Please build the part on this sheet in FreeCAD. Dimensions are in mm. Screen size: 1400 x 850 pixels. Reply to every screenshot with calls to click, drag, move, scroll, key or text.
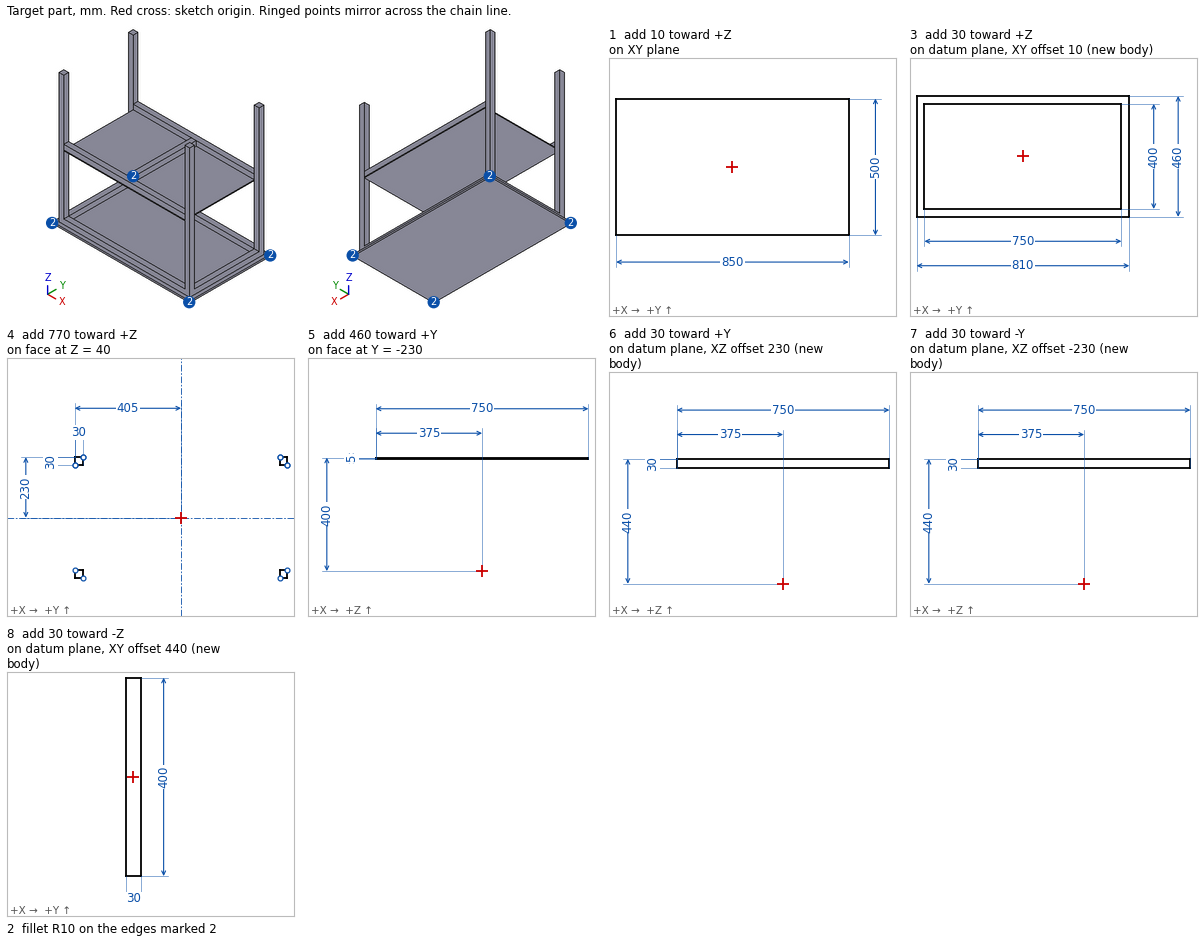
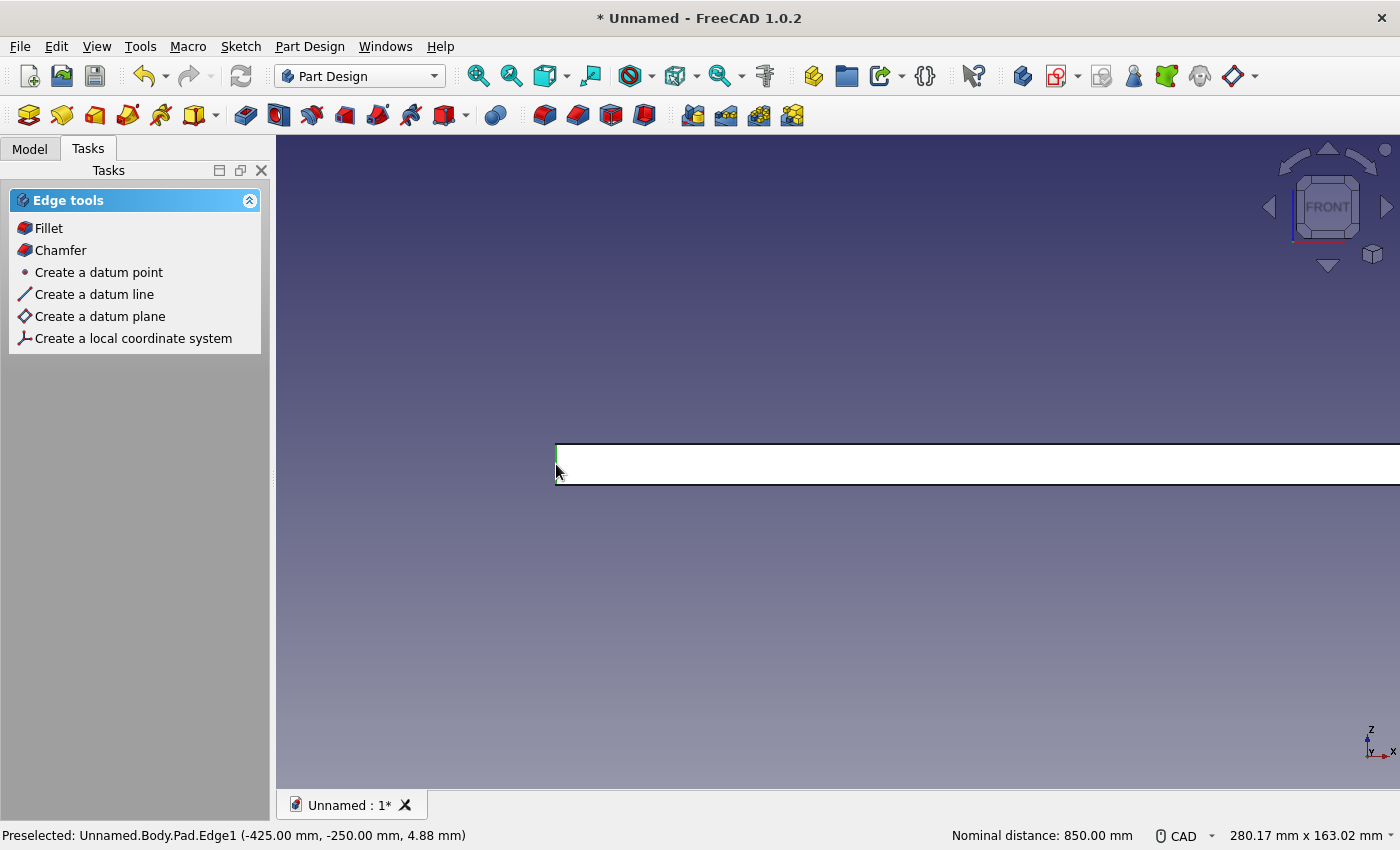
click(479, 76)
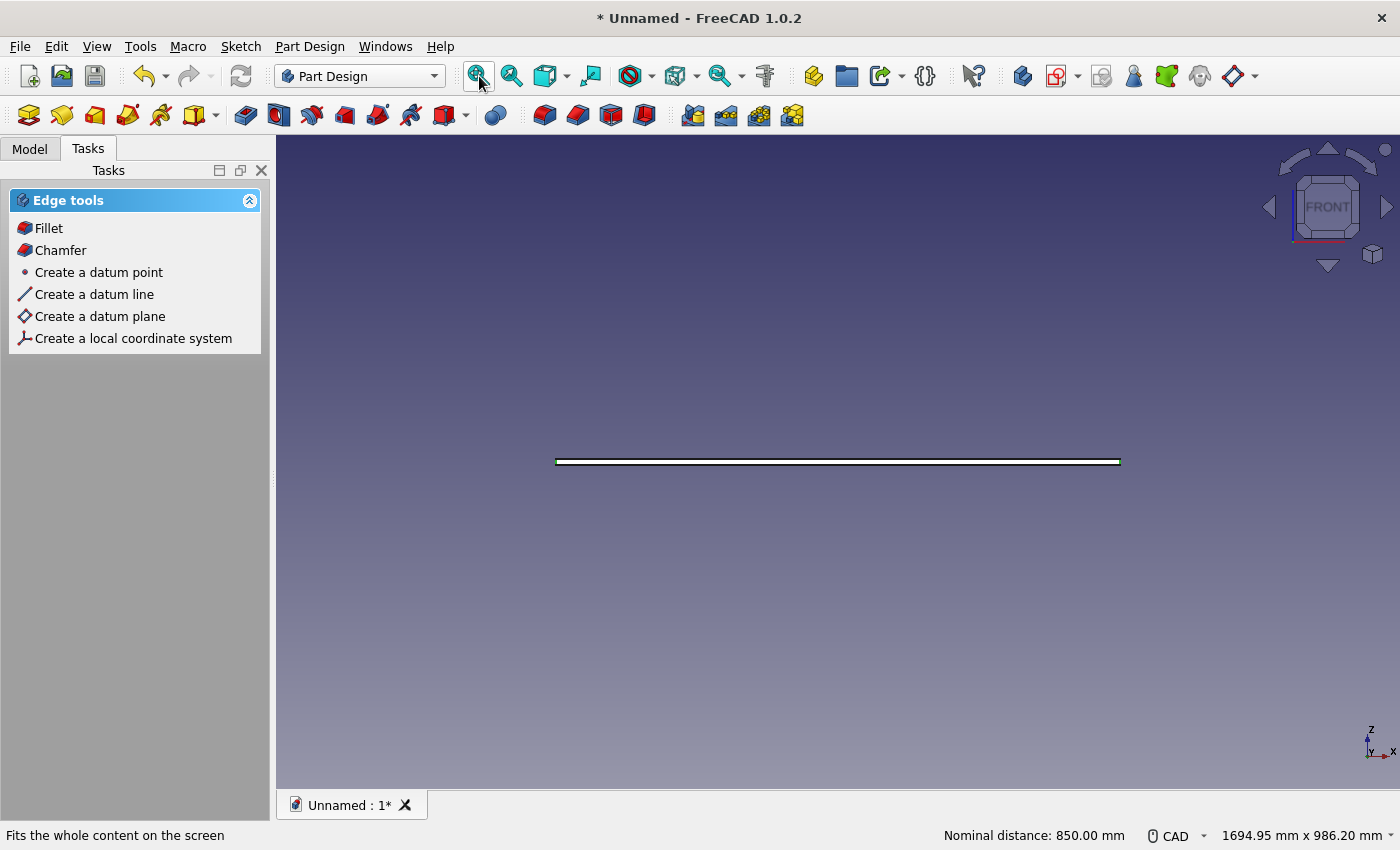
key(3)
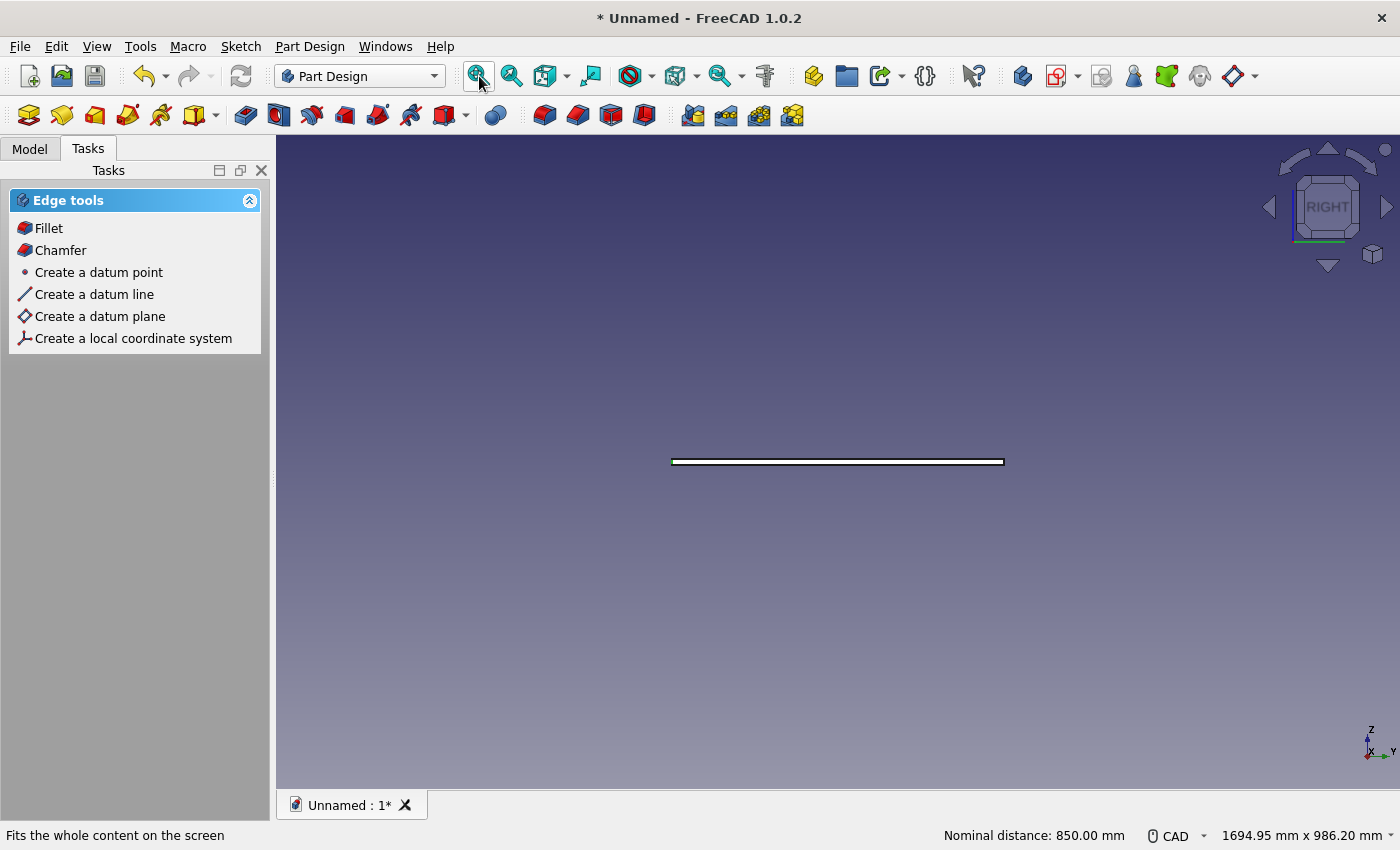
click(479, 76)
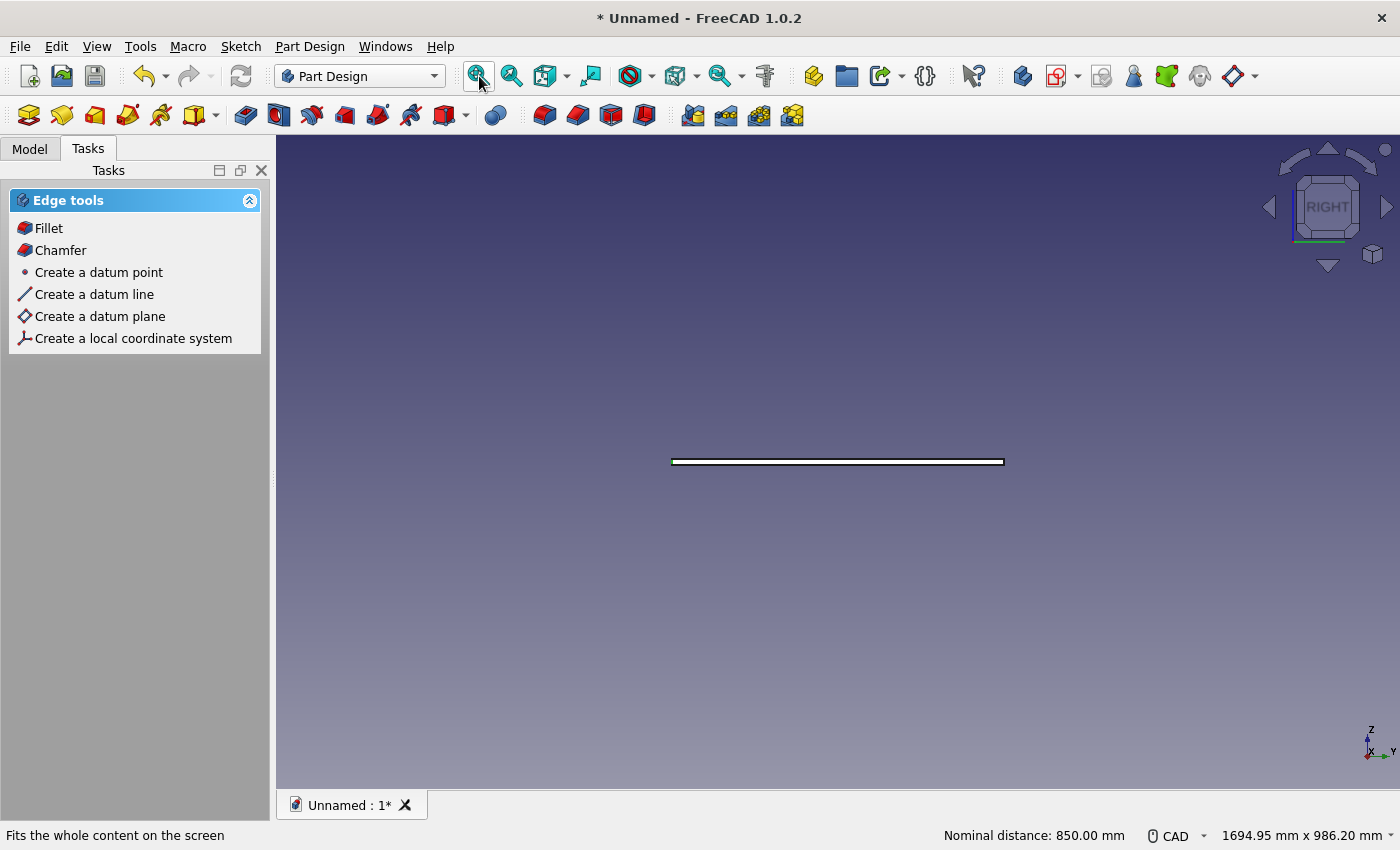
scroll(1004, 461, up, 9)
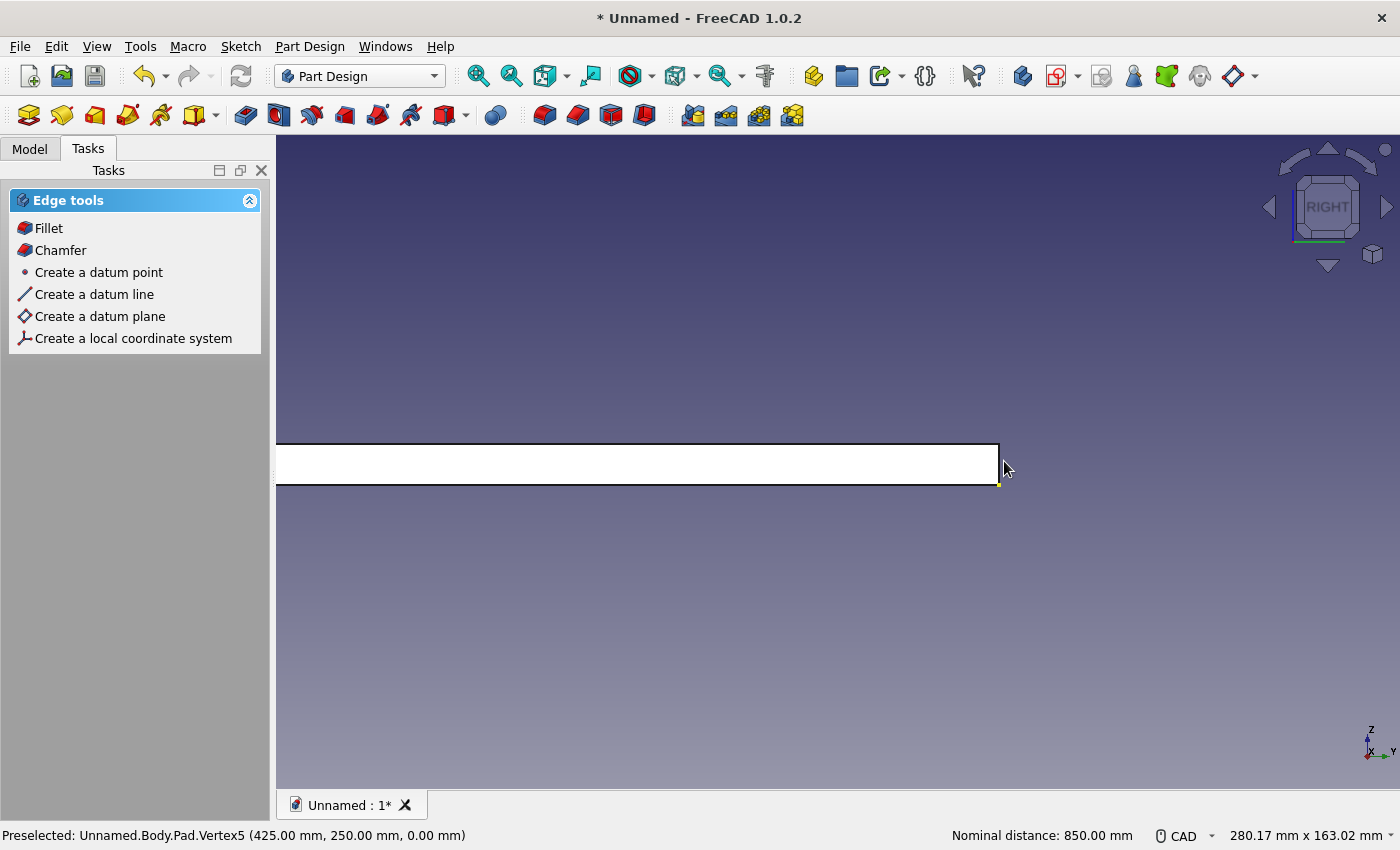
click(999, 464, ctrl)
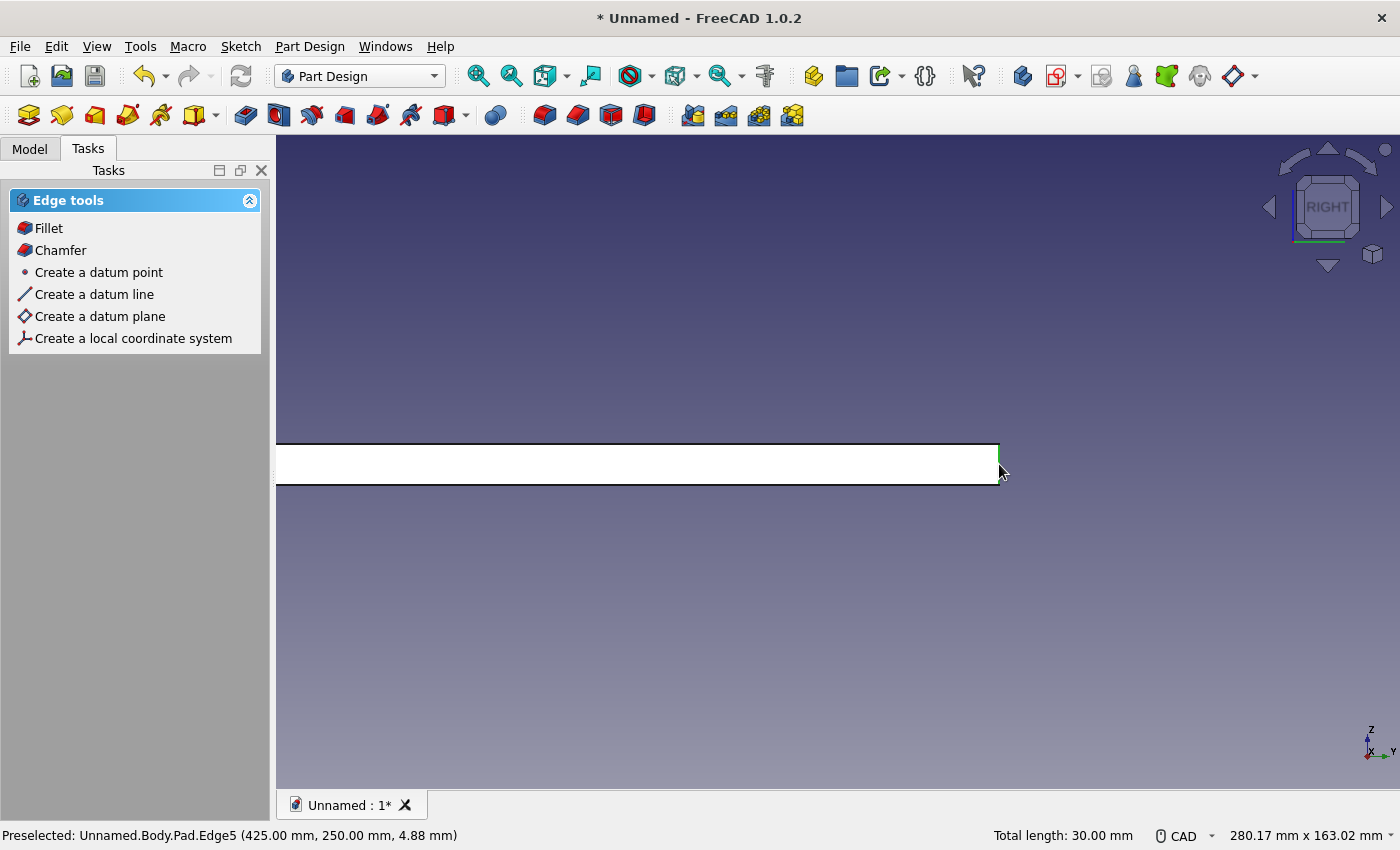
click(479, 76)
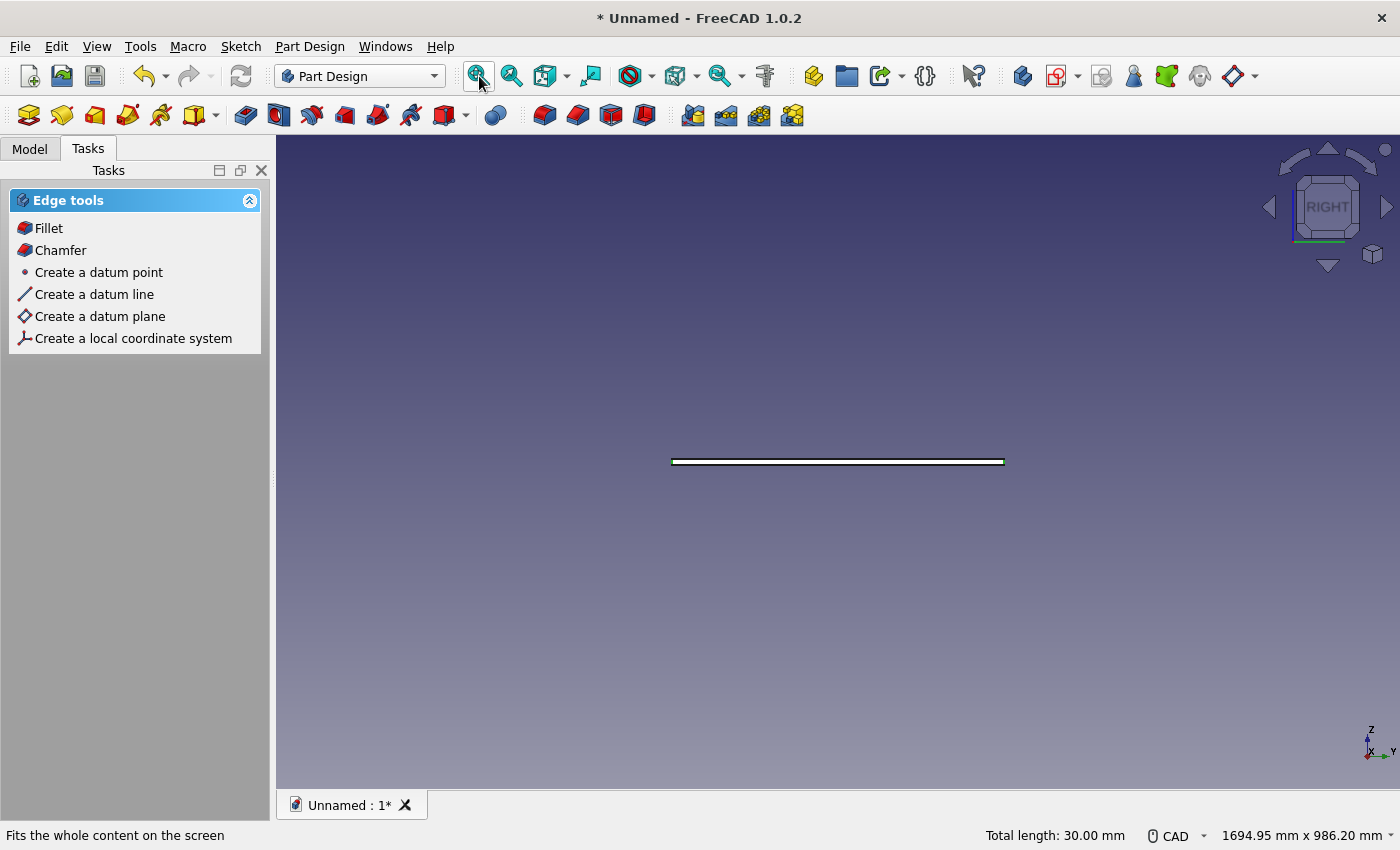
key(5)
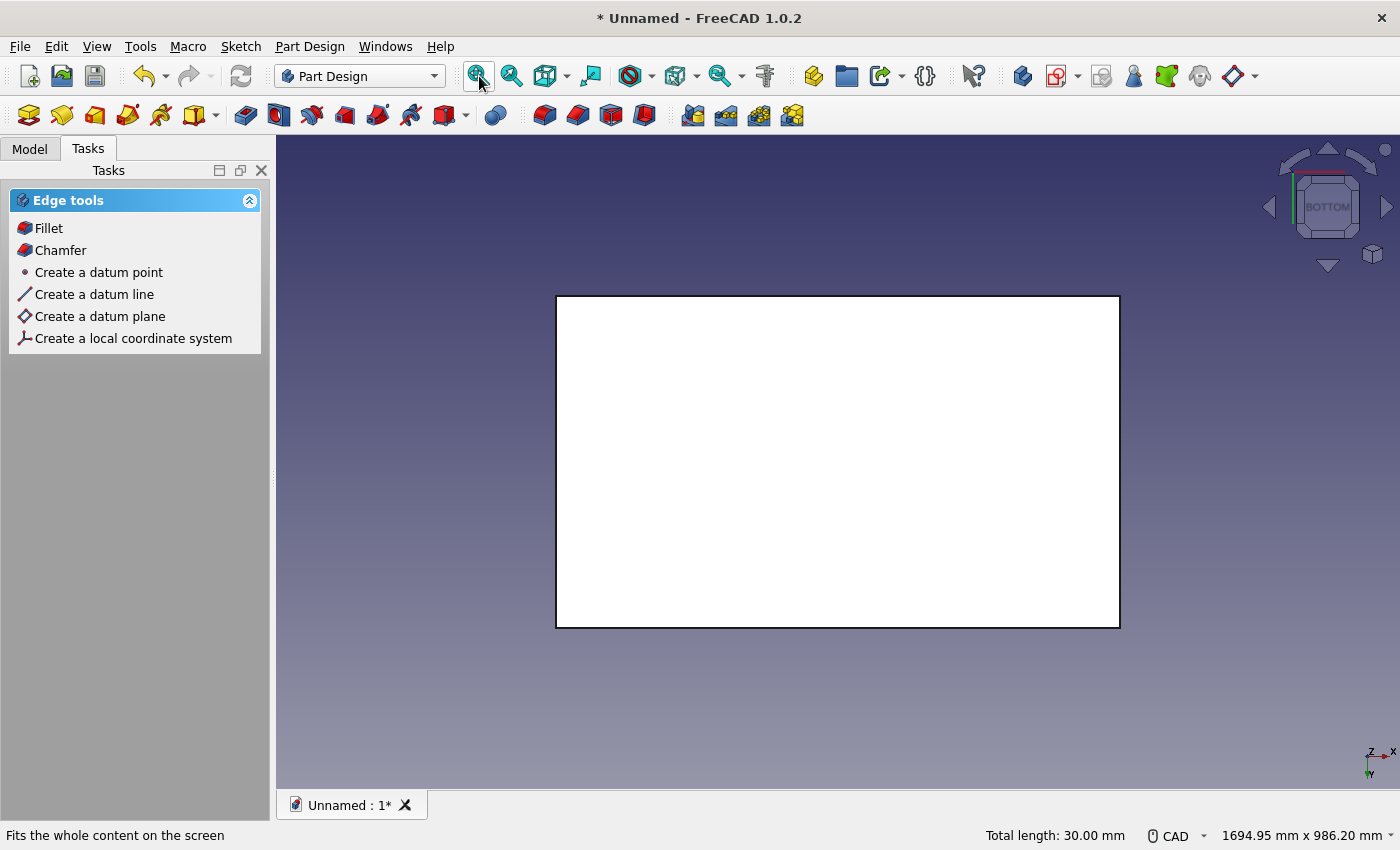
scroll(556, 627, up, 9)